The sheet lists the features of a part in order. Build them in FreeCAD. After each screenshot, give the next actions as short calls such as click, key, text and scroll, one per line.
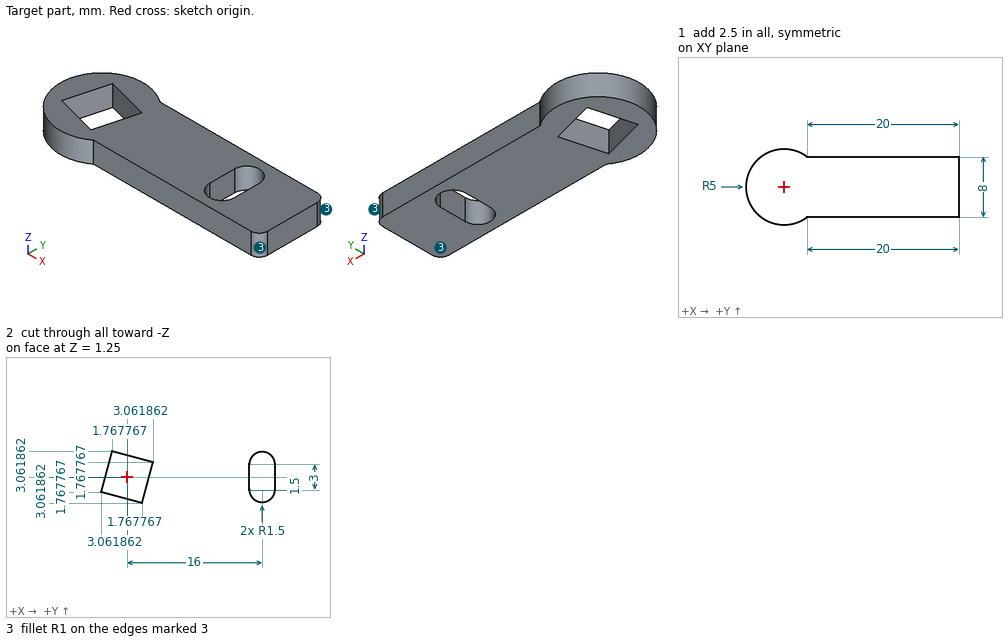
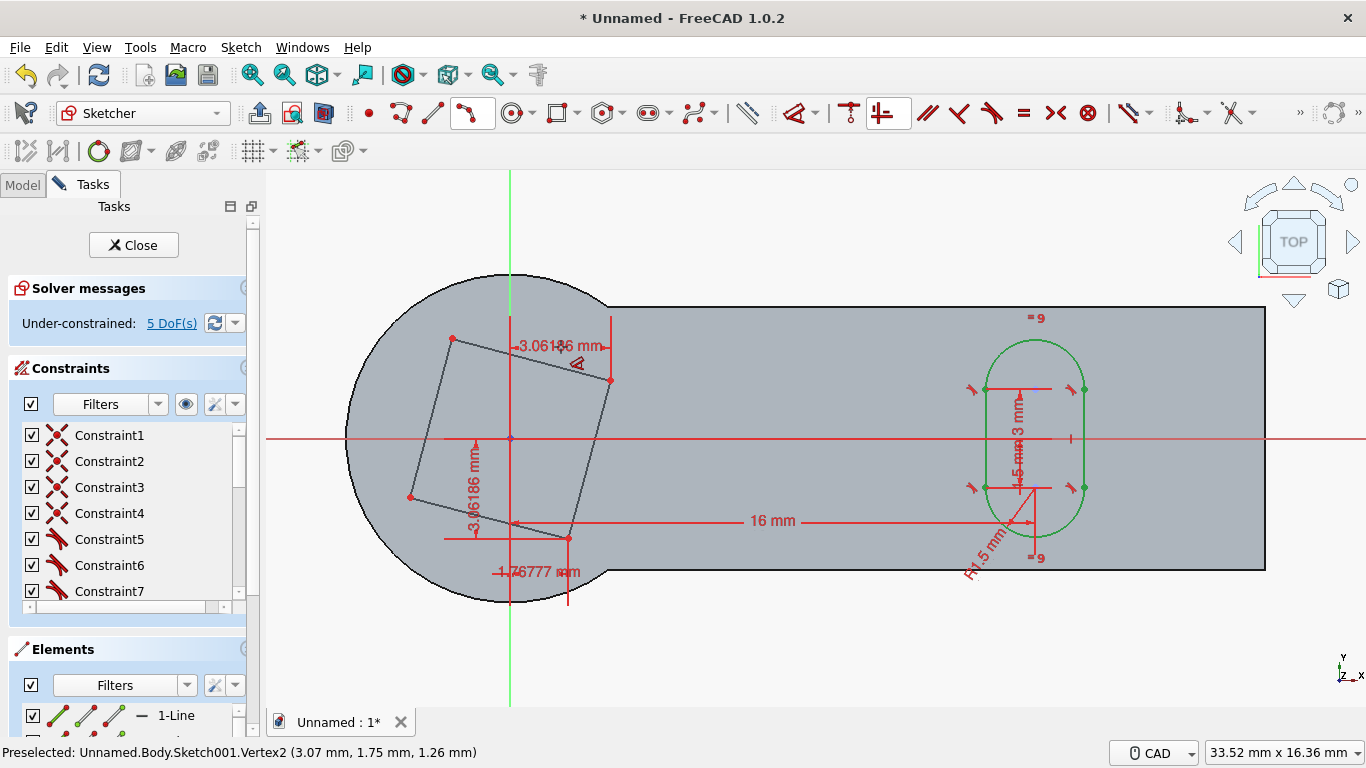
click(611, 381)
click(476, 410)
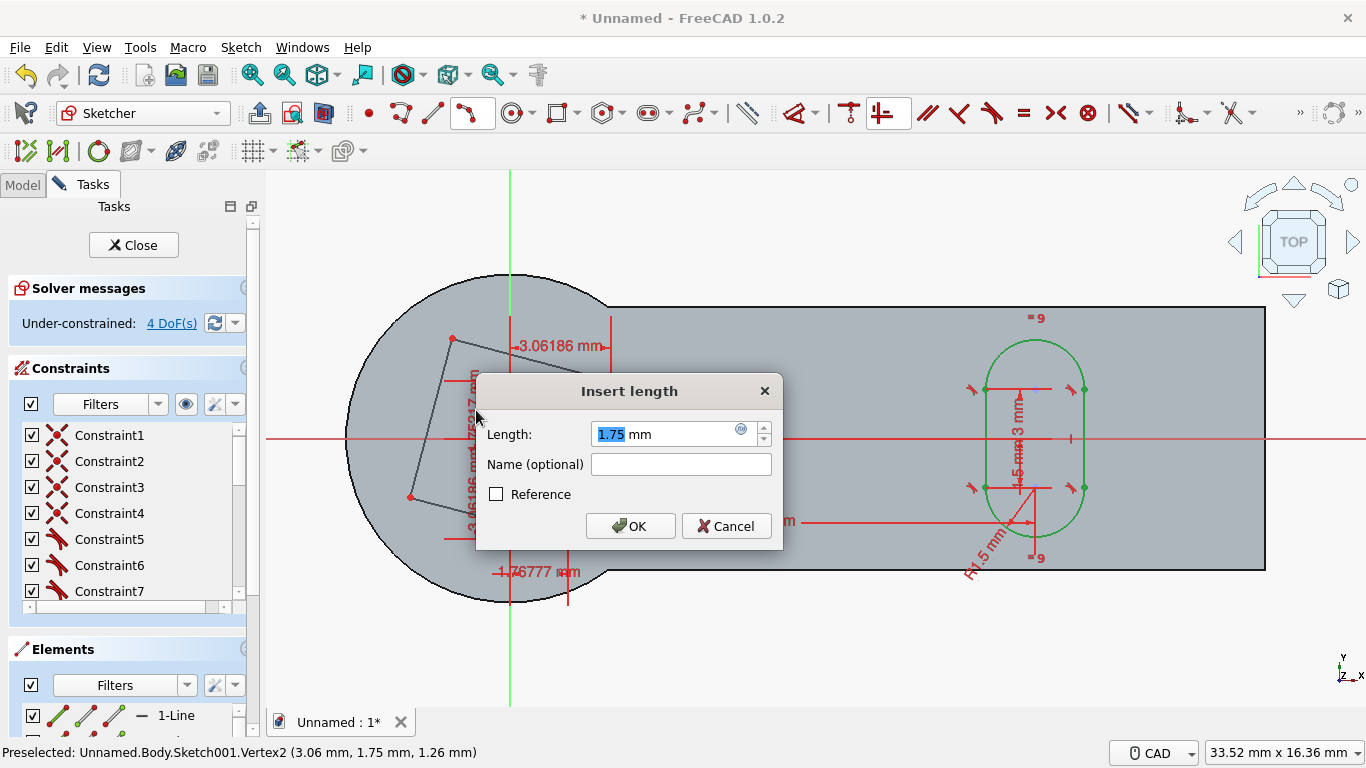
text(1.767767)
key(Return)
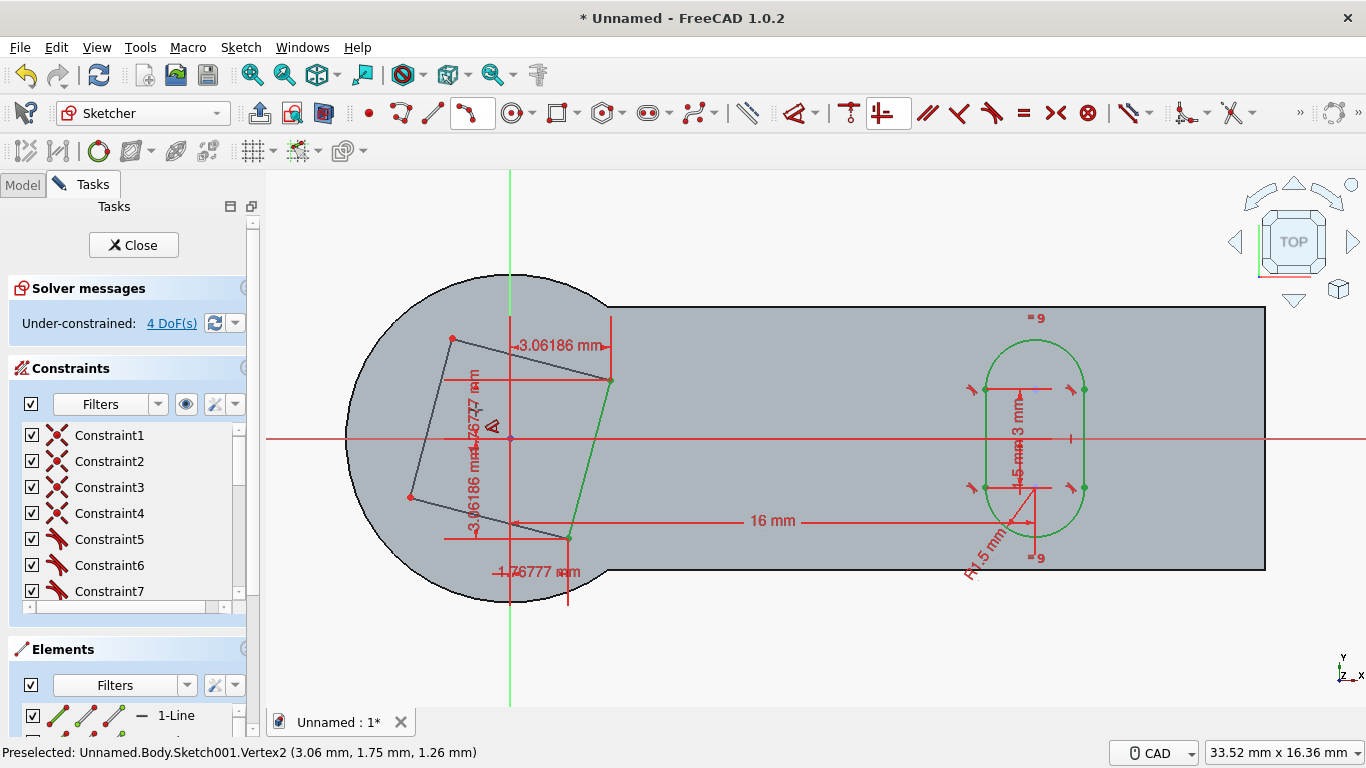
click(452, 339)
click(481, 305)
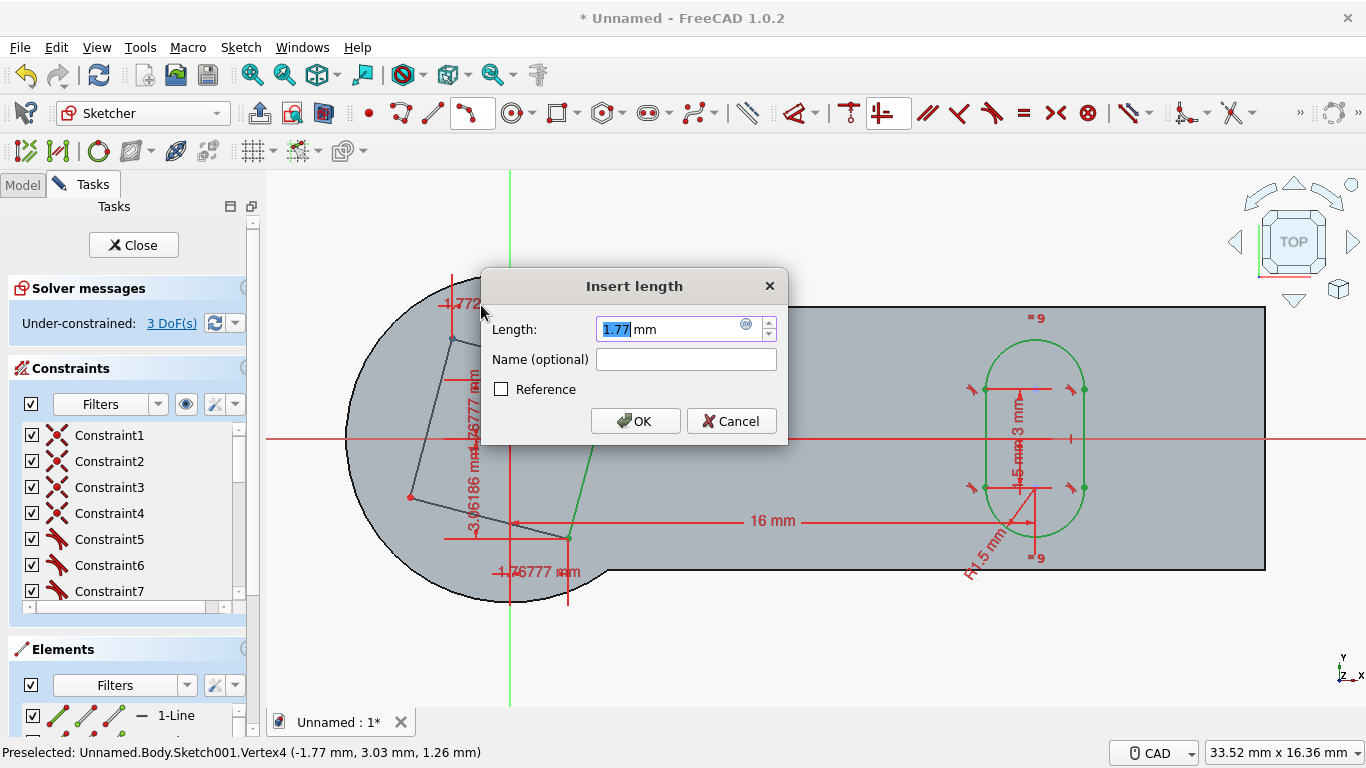
text(1.767767)
key(Return)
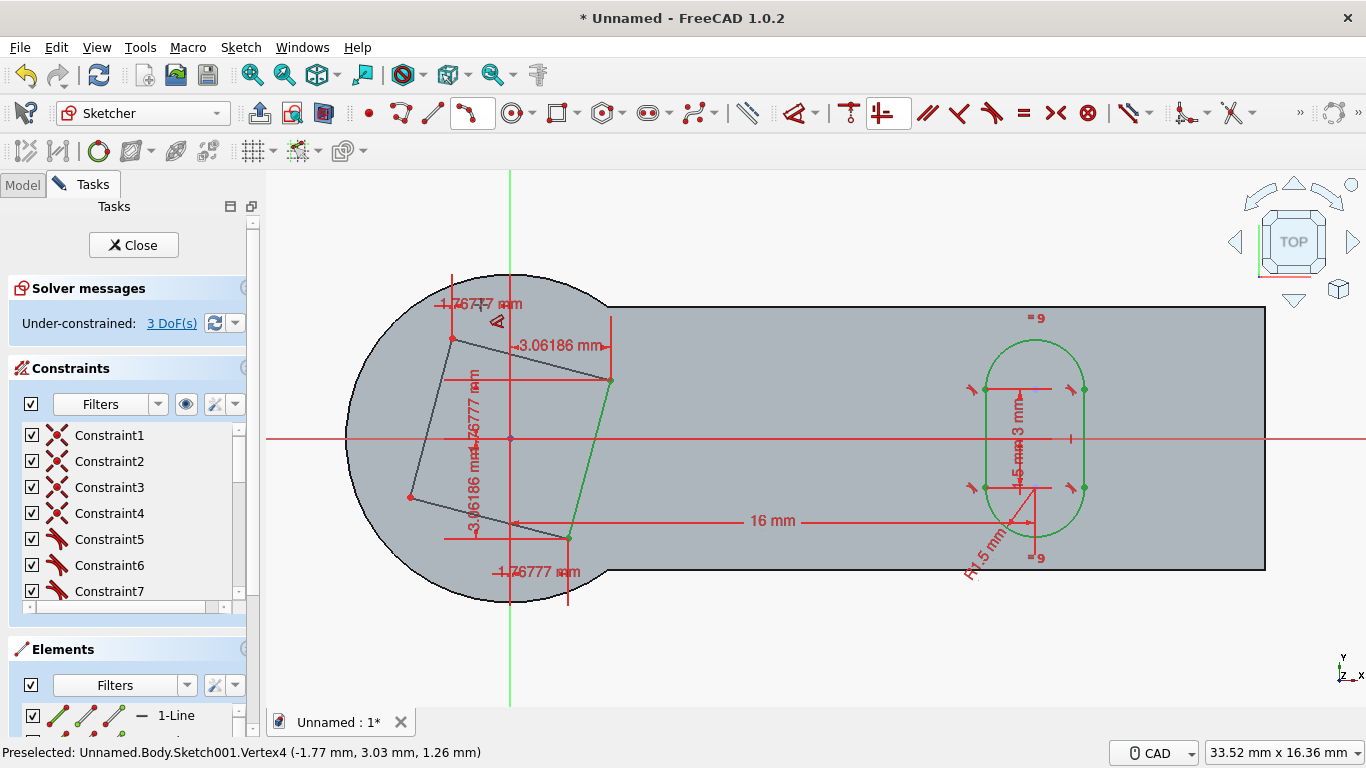
click(452, 339)
click(418, 389)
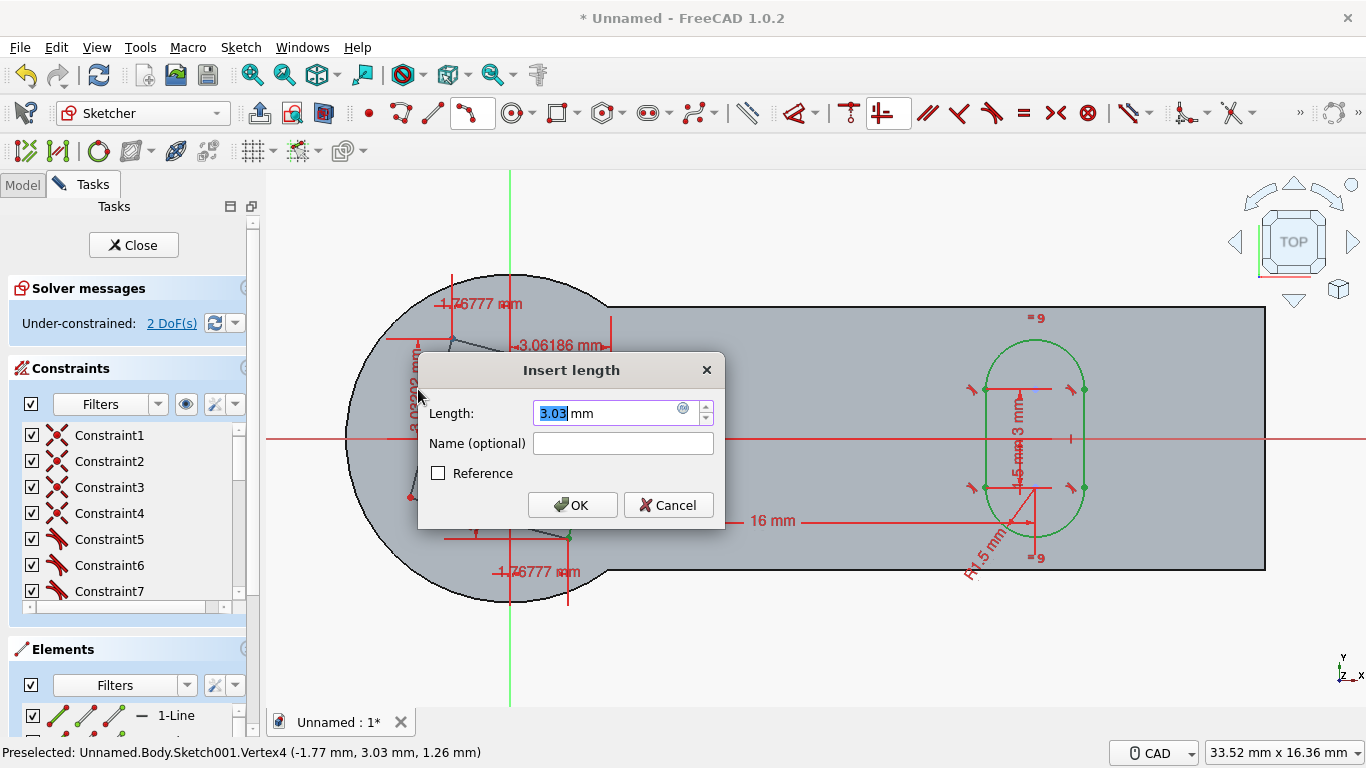
text(3.061862)
key(Return)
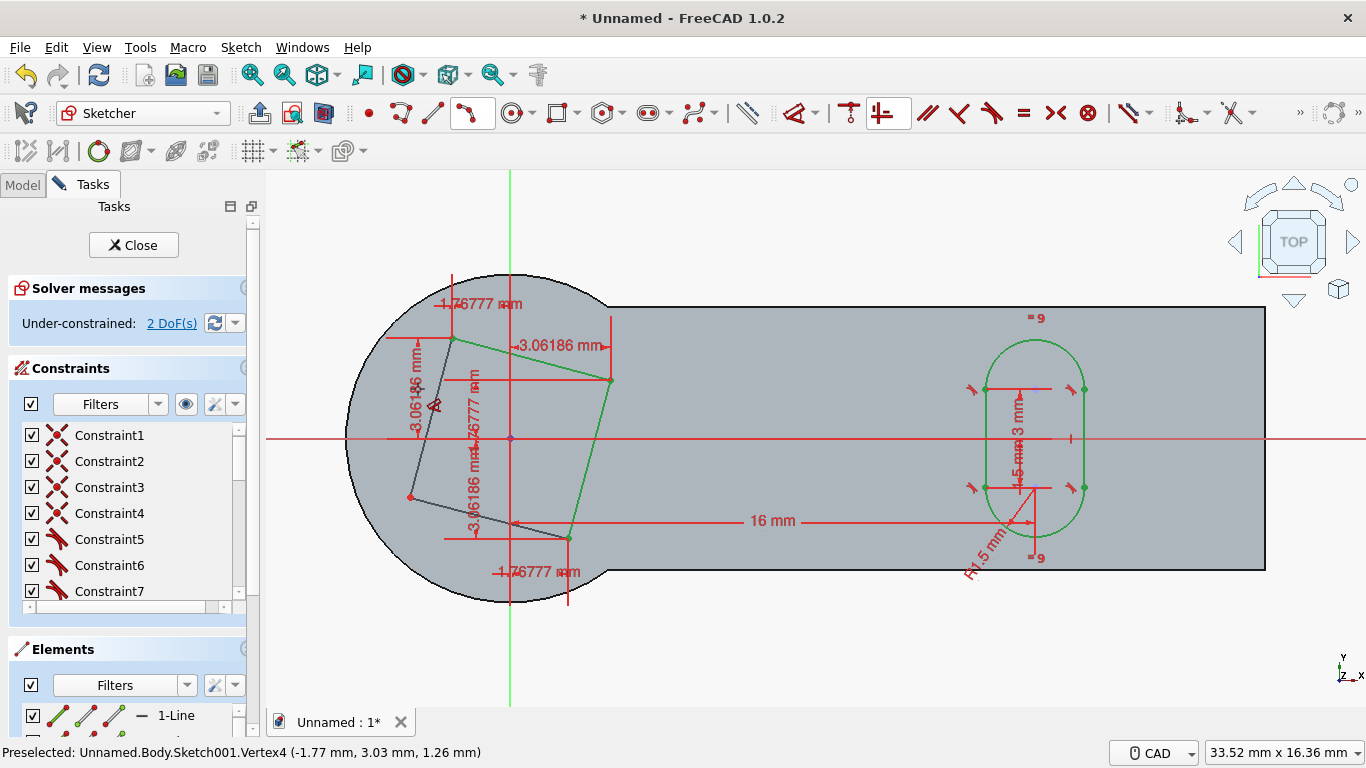
click(410, 498)
click(460, 532)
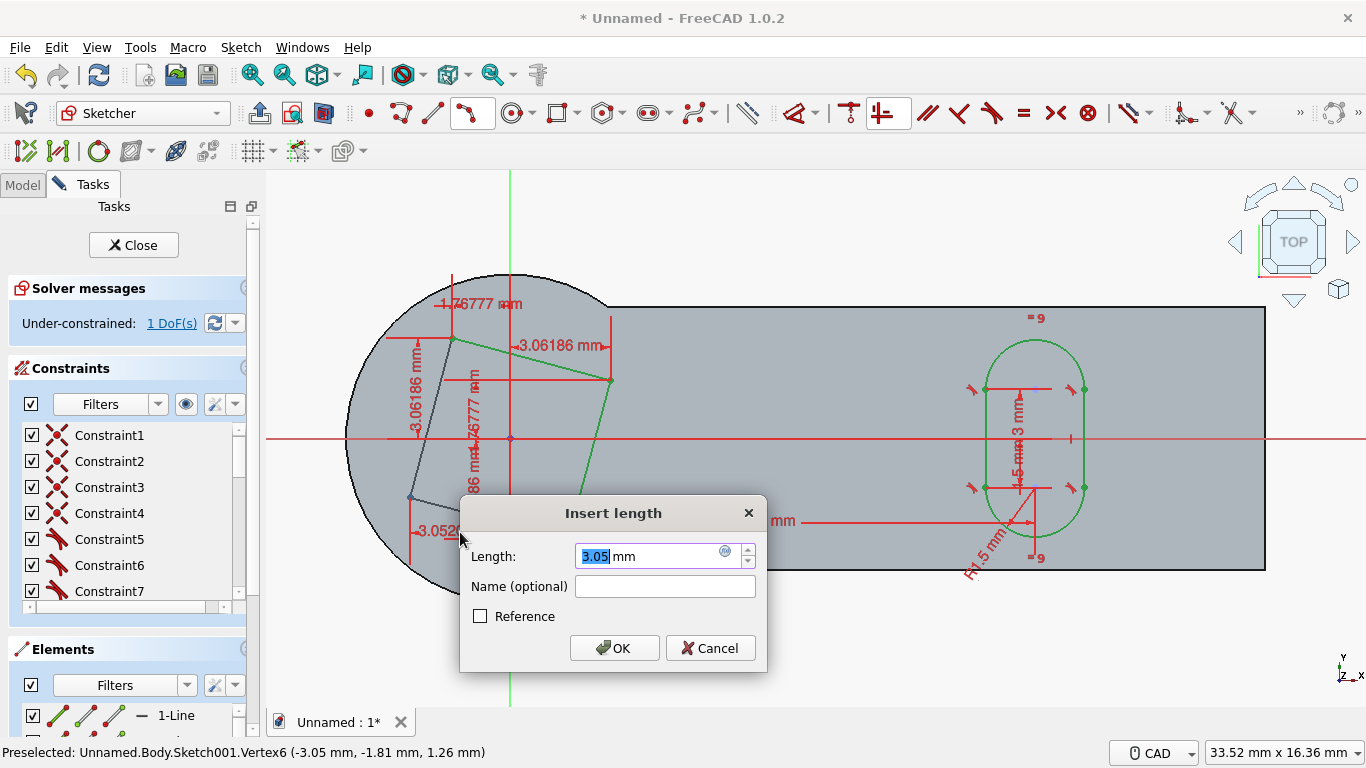
text(3.061862)
key(Return)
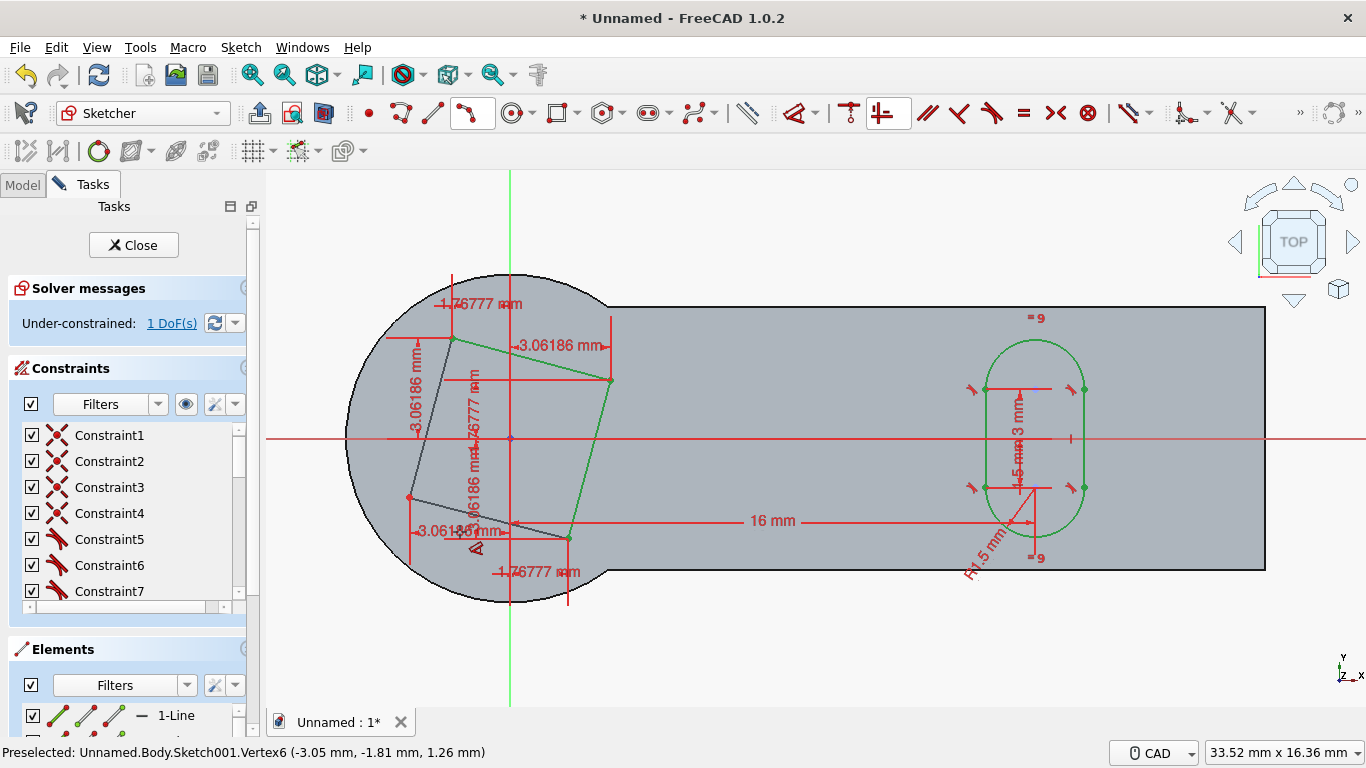
click(410, 498)
click(376, 468)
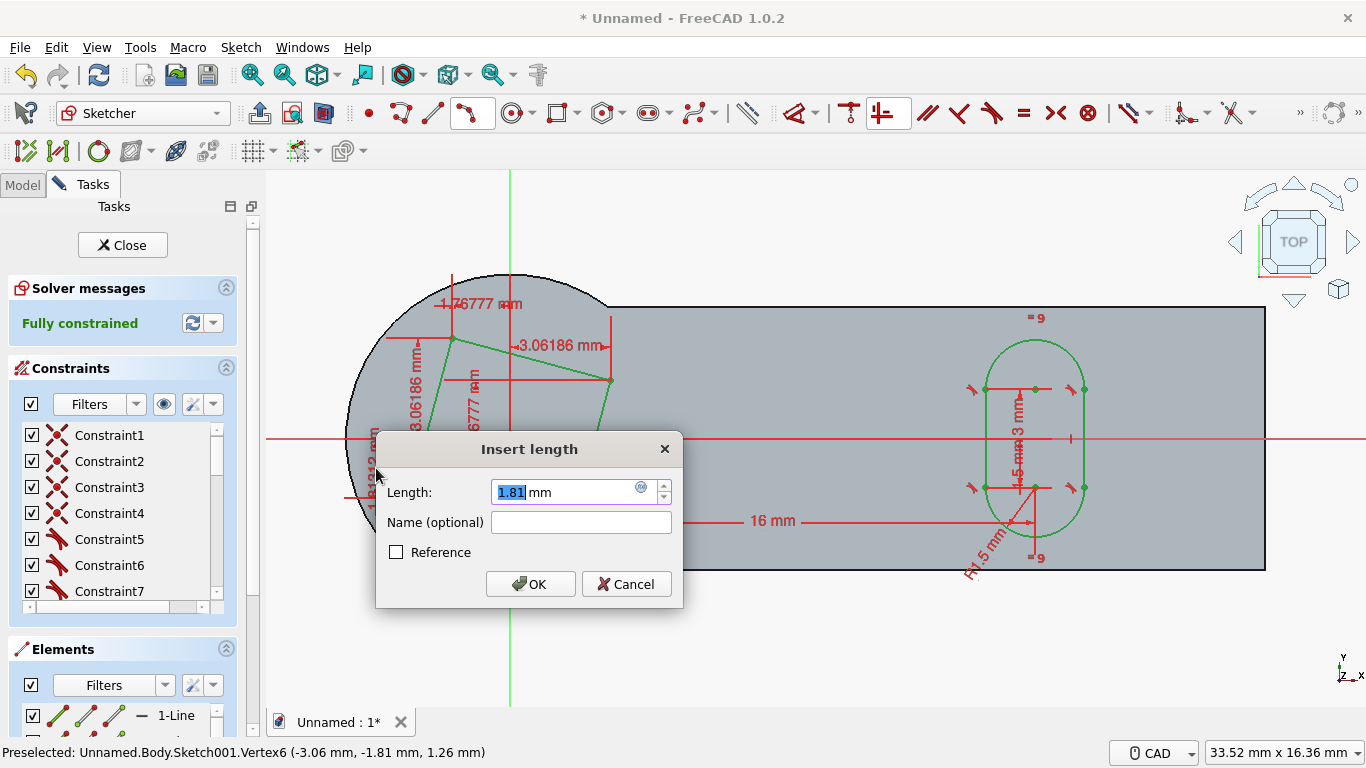
text(1.767767)
key(Return)
key(Escape)